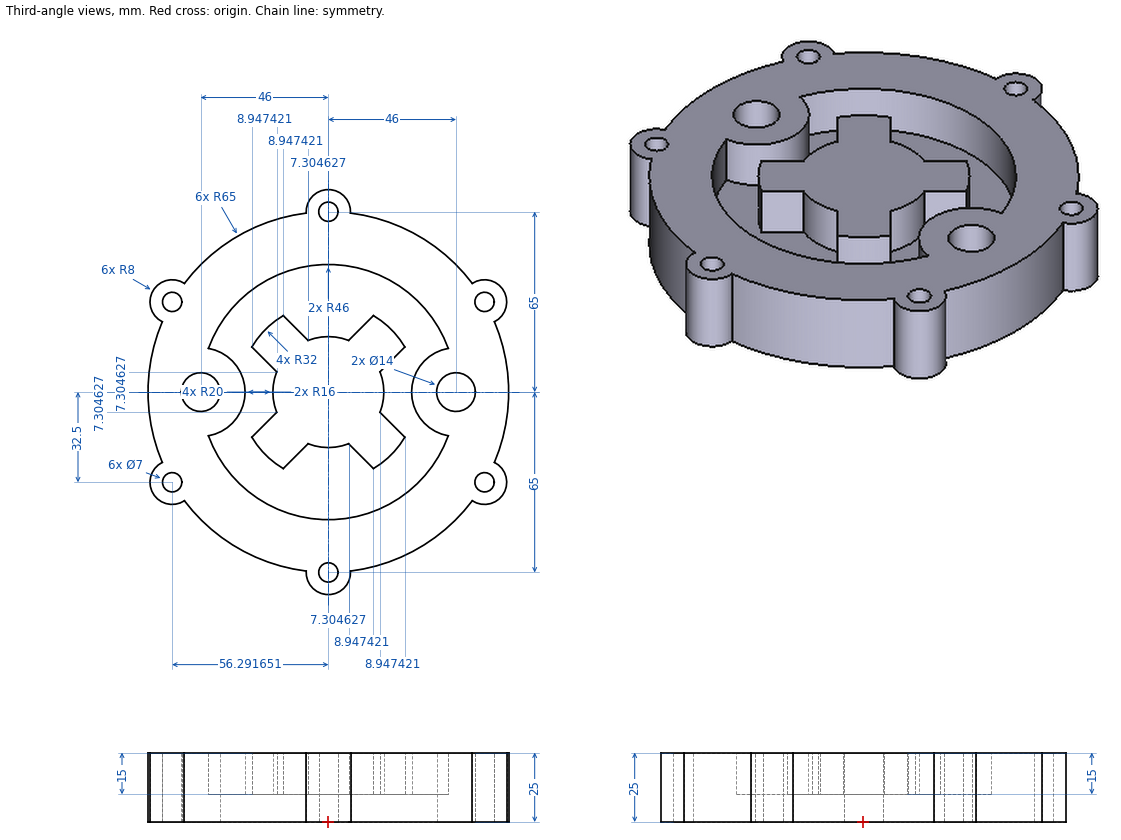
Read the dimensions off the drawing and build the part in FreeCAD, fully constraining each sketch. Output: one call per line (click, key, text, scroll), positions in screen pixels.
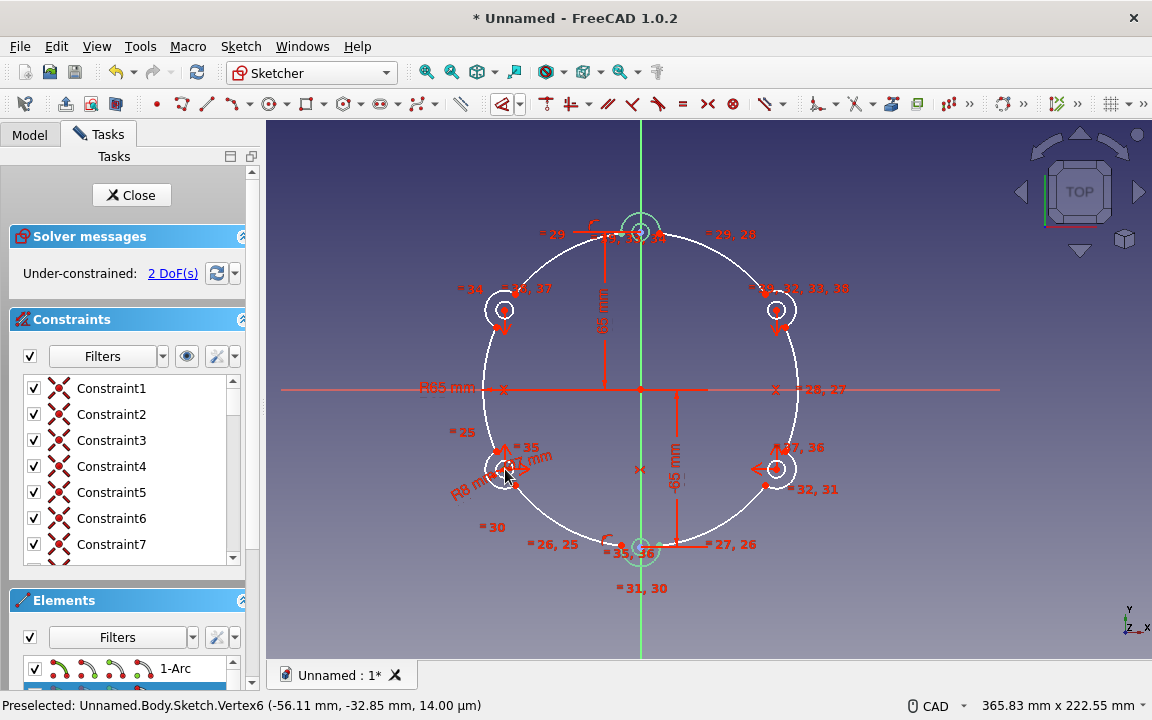
click(520, 104)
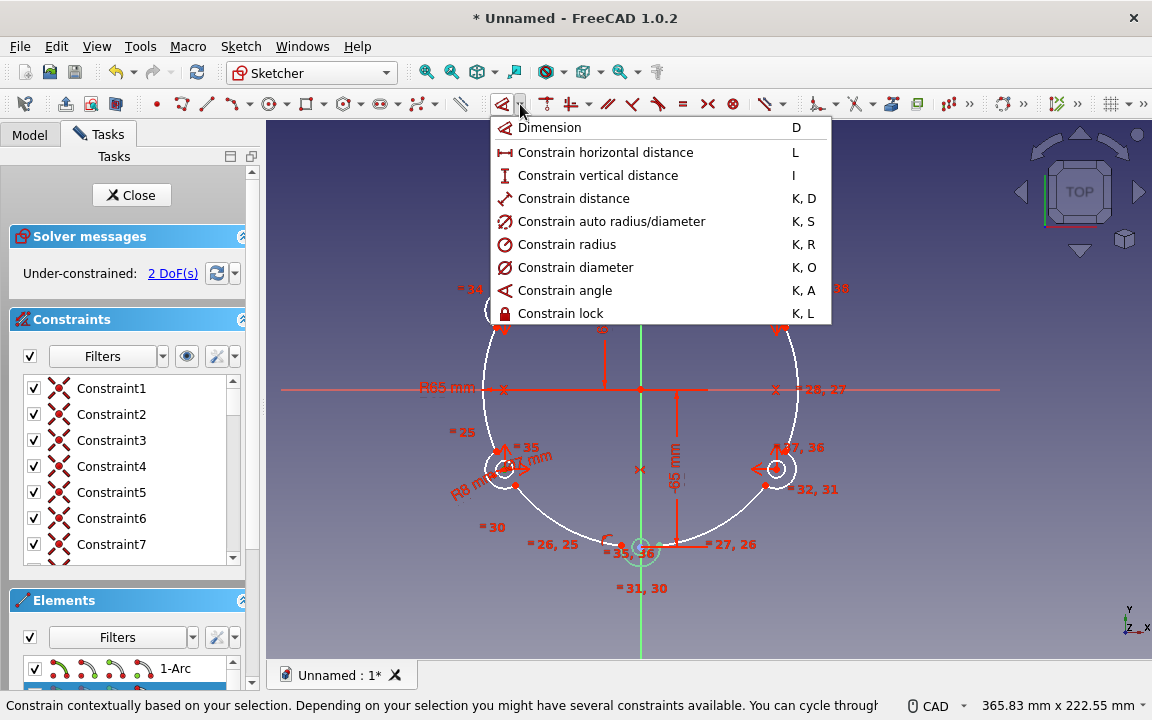
click(661, 176)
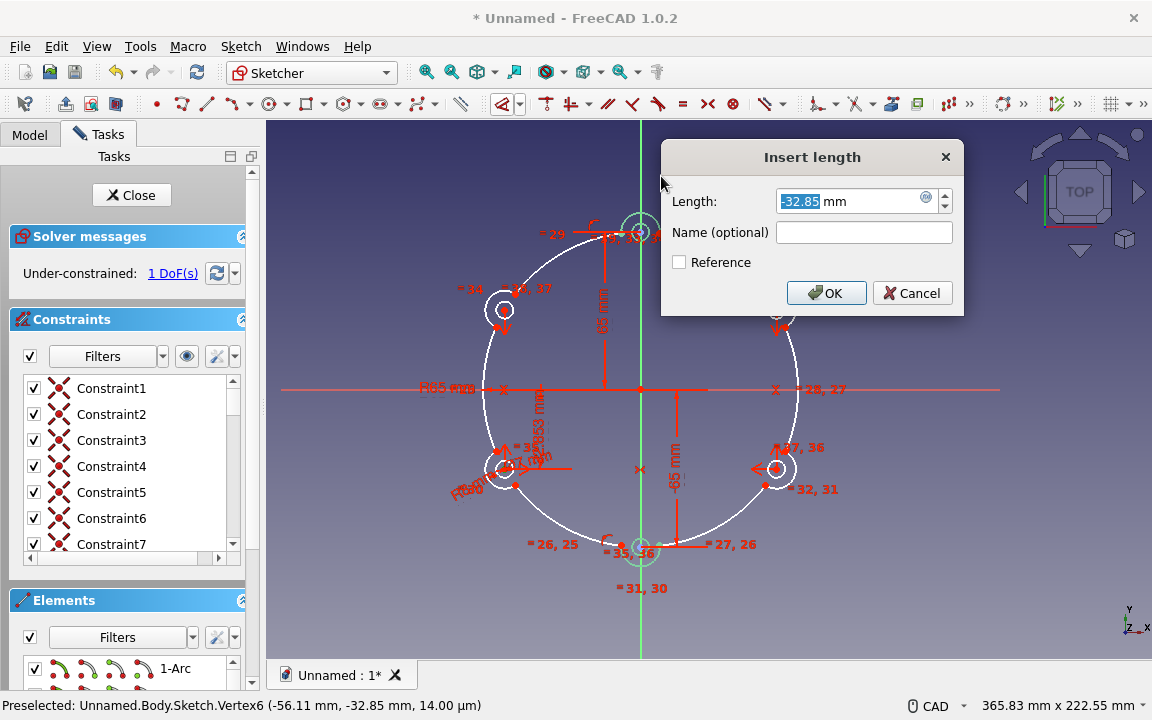
text(-32.5)
key(Return)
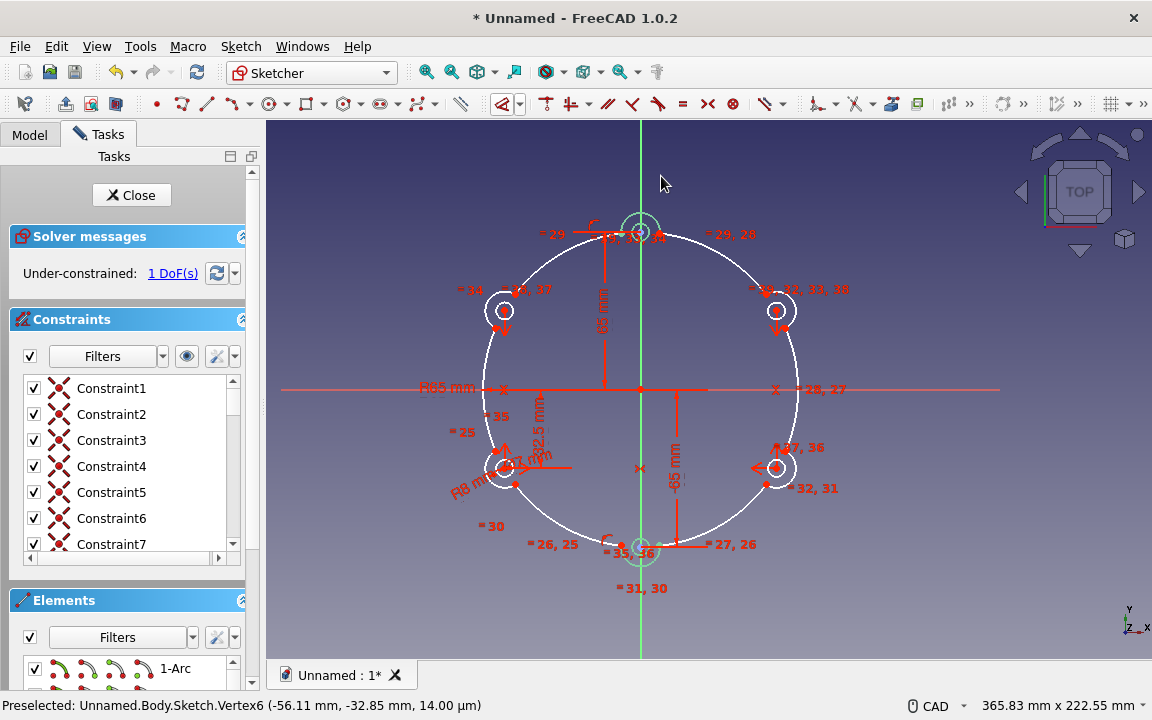
click(505, 468)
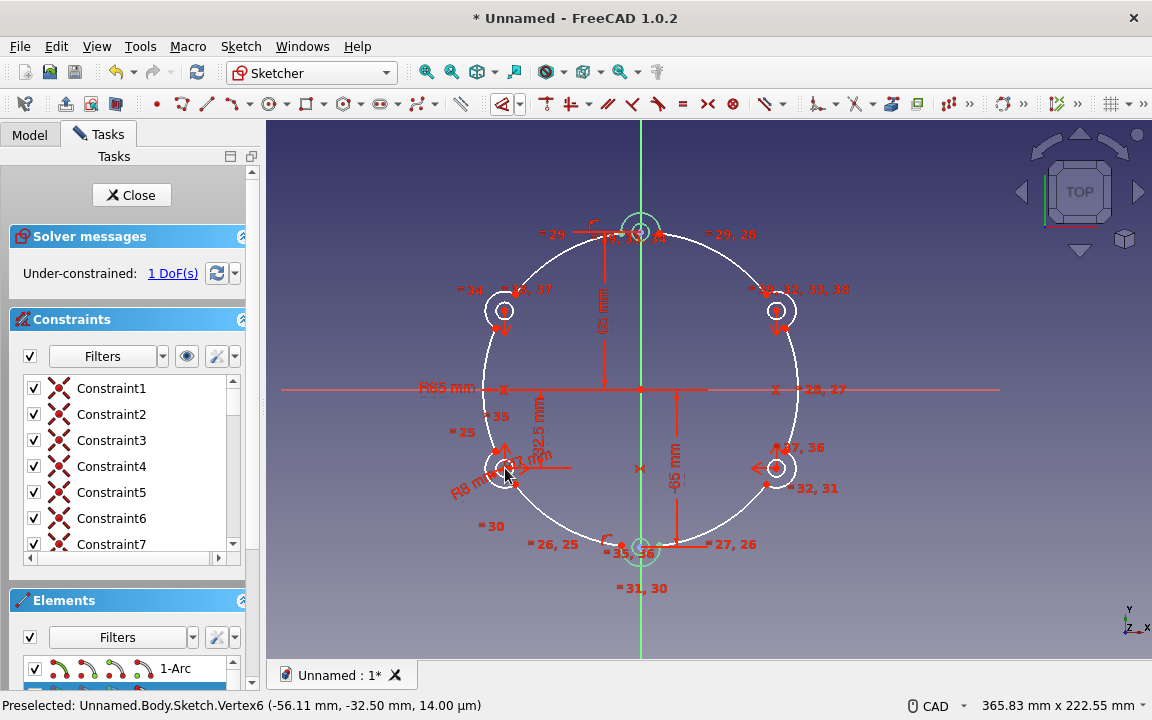
key(l)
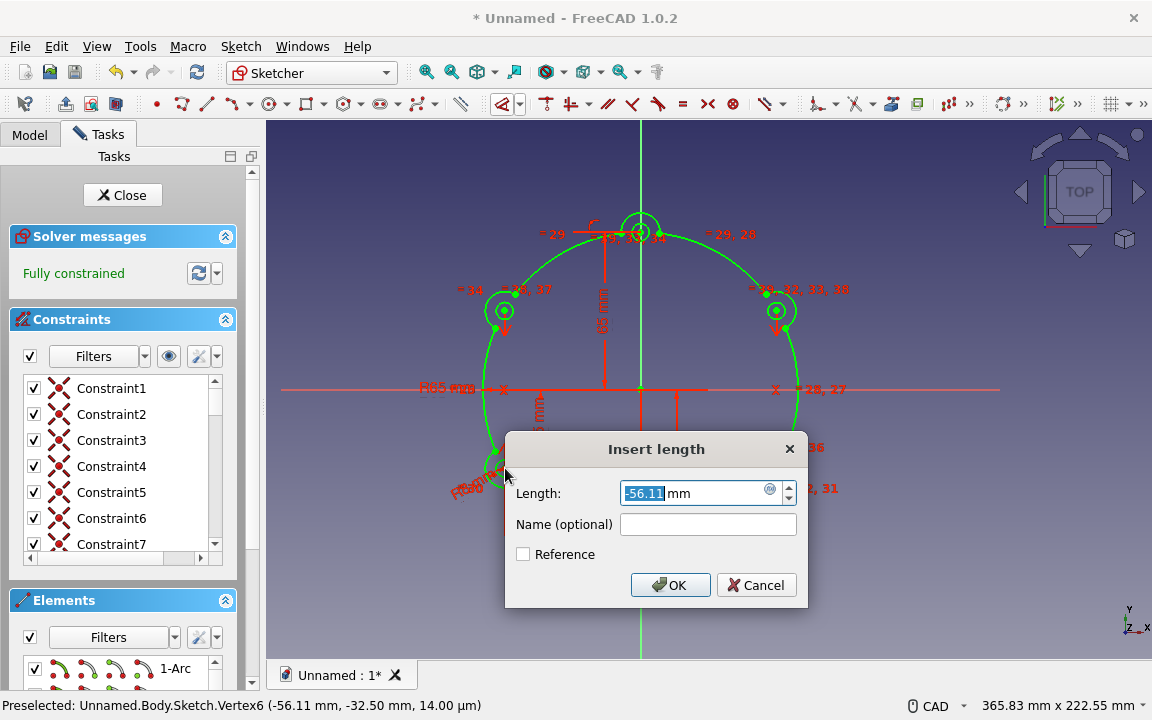
text(-56.291651)
key(Return)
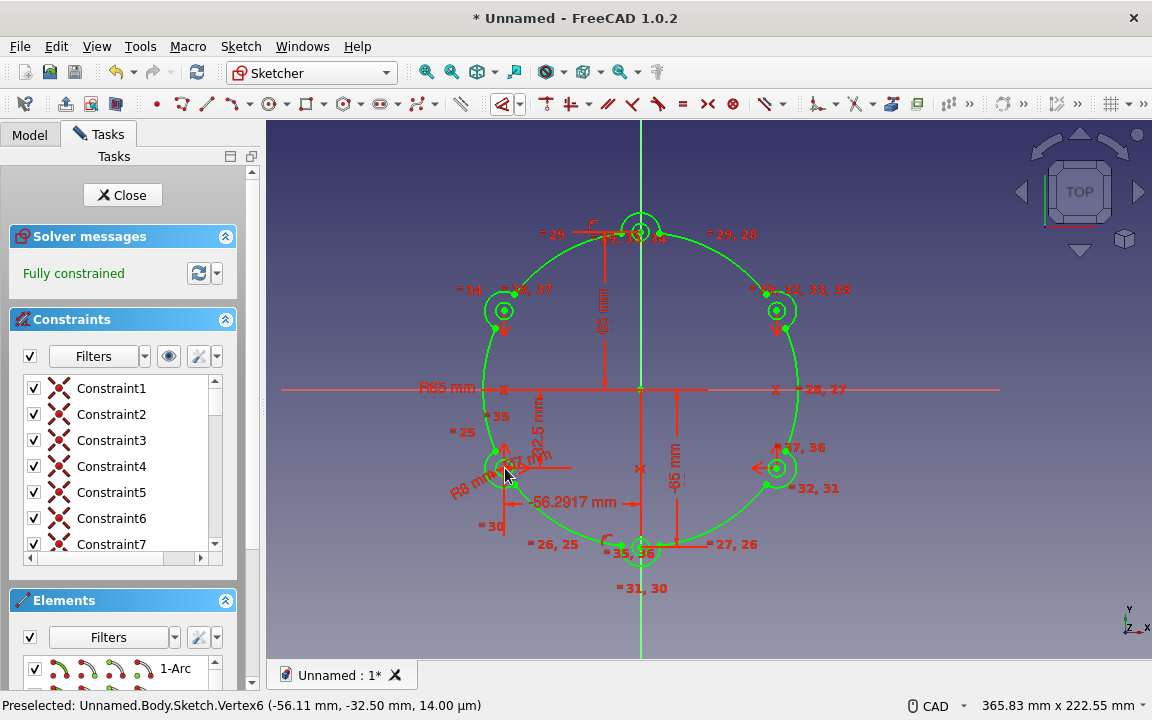
click(123, 195)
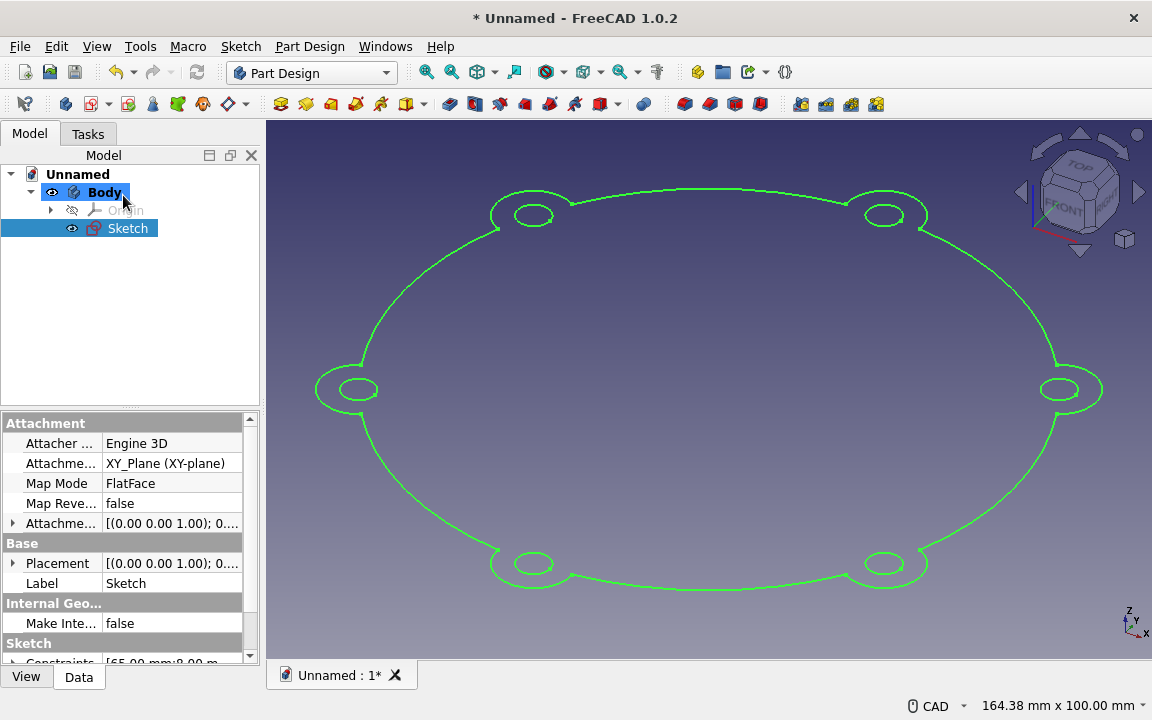
click(281, 104)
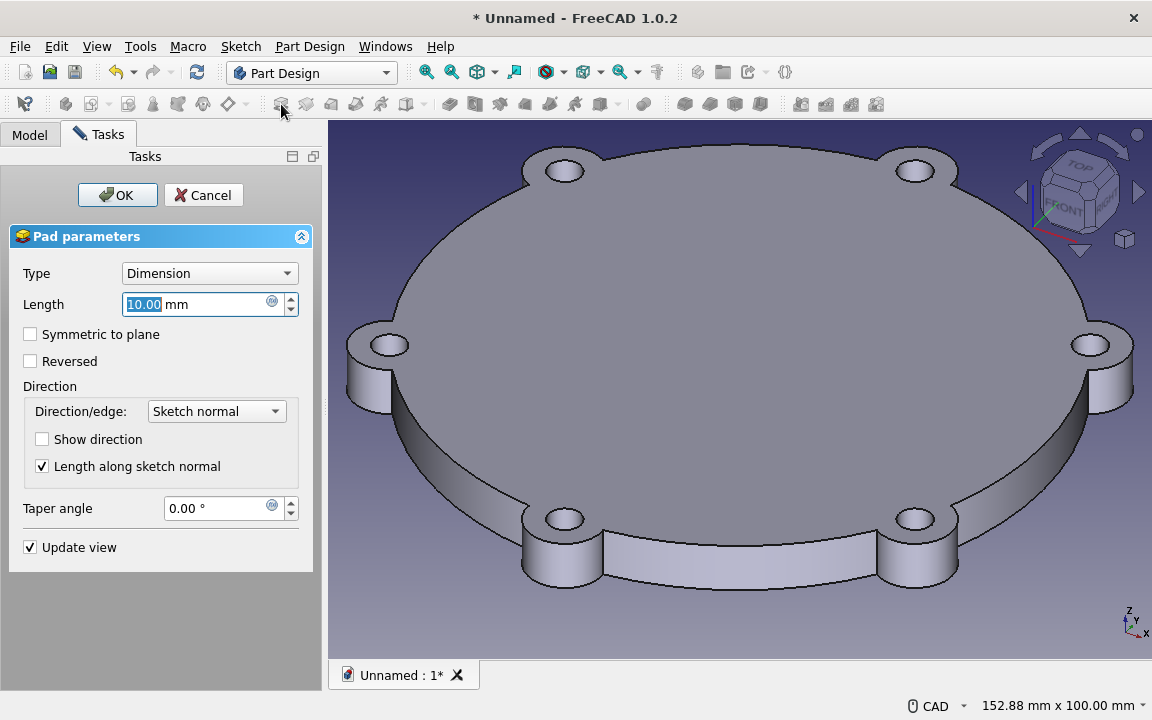
text(25)
key(Tab)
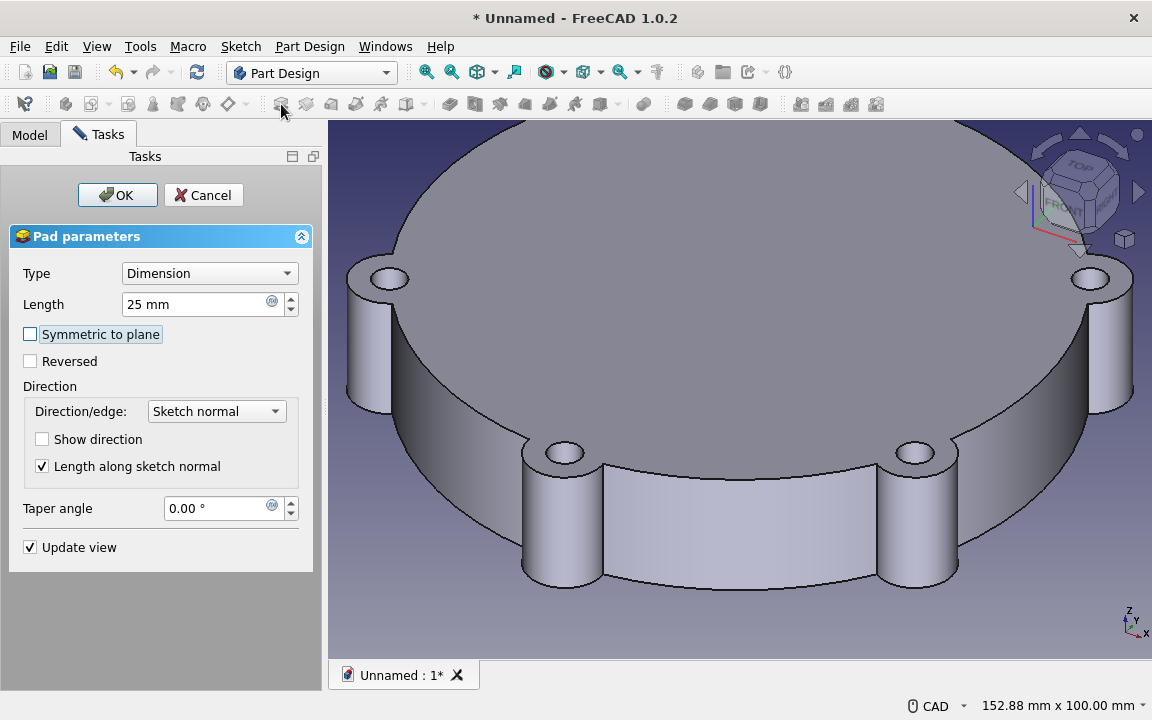
click(118, 195)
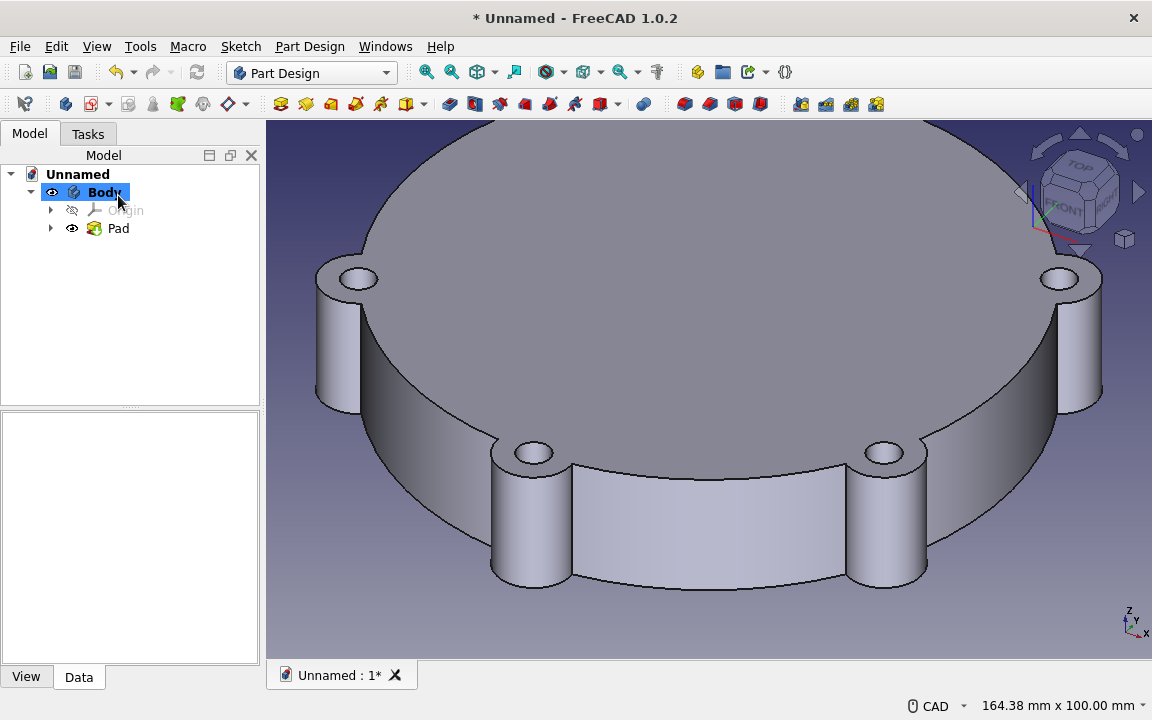
click(427, 72)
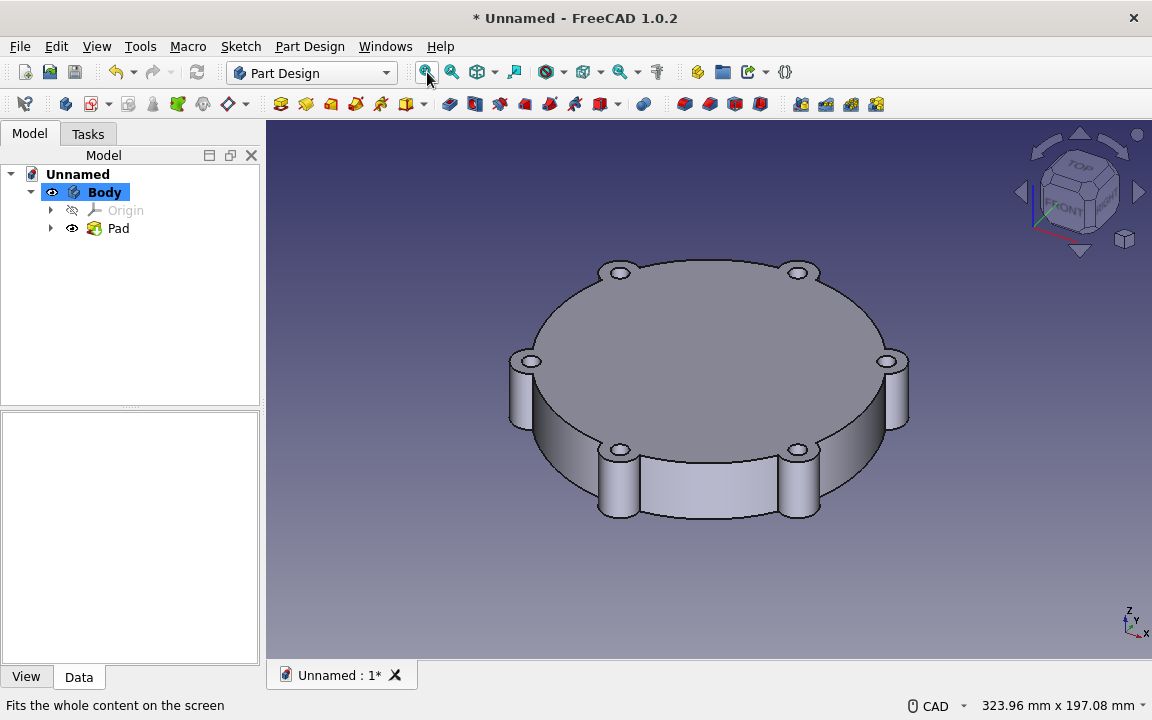
click(709, 360)